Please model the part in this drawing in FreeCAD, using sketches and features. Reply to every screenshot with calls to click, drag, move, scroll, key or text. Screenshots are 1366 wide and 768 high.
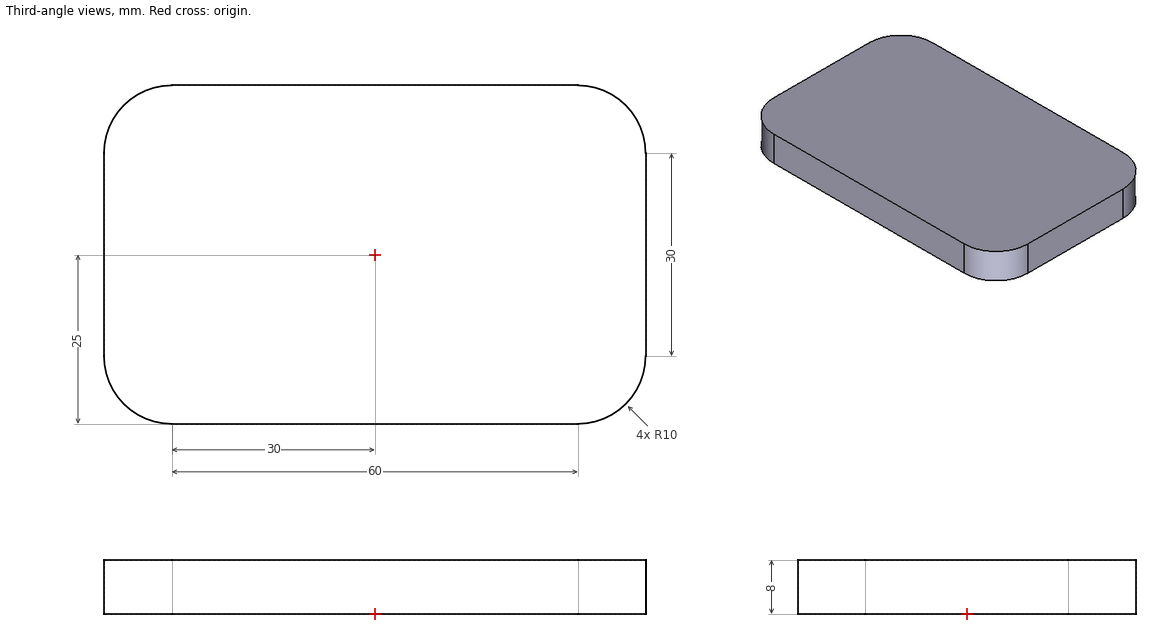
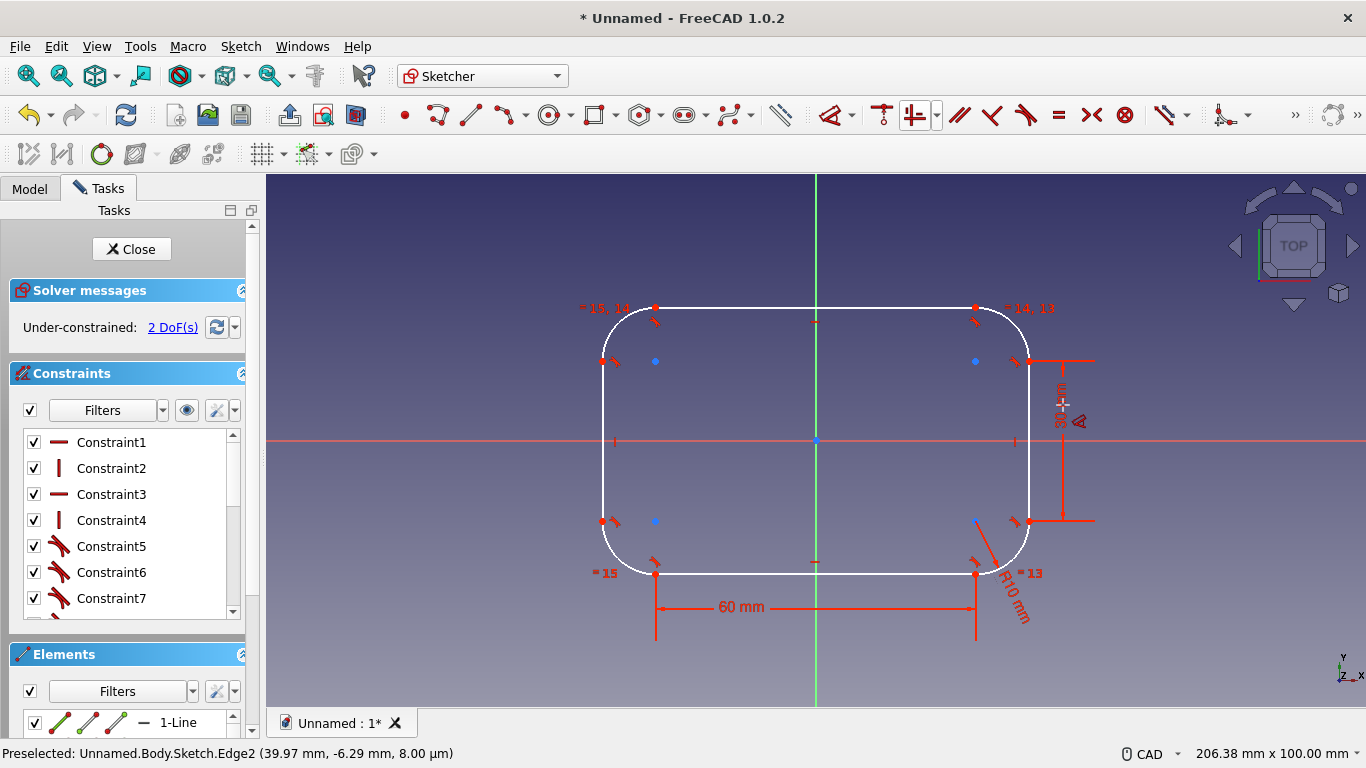
click(656, 574)
click(736, 406)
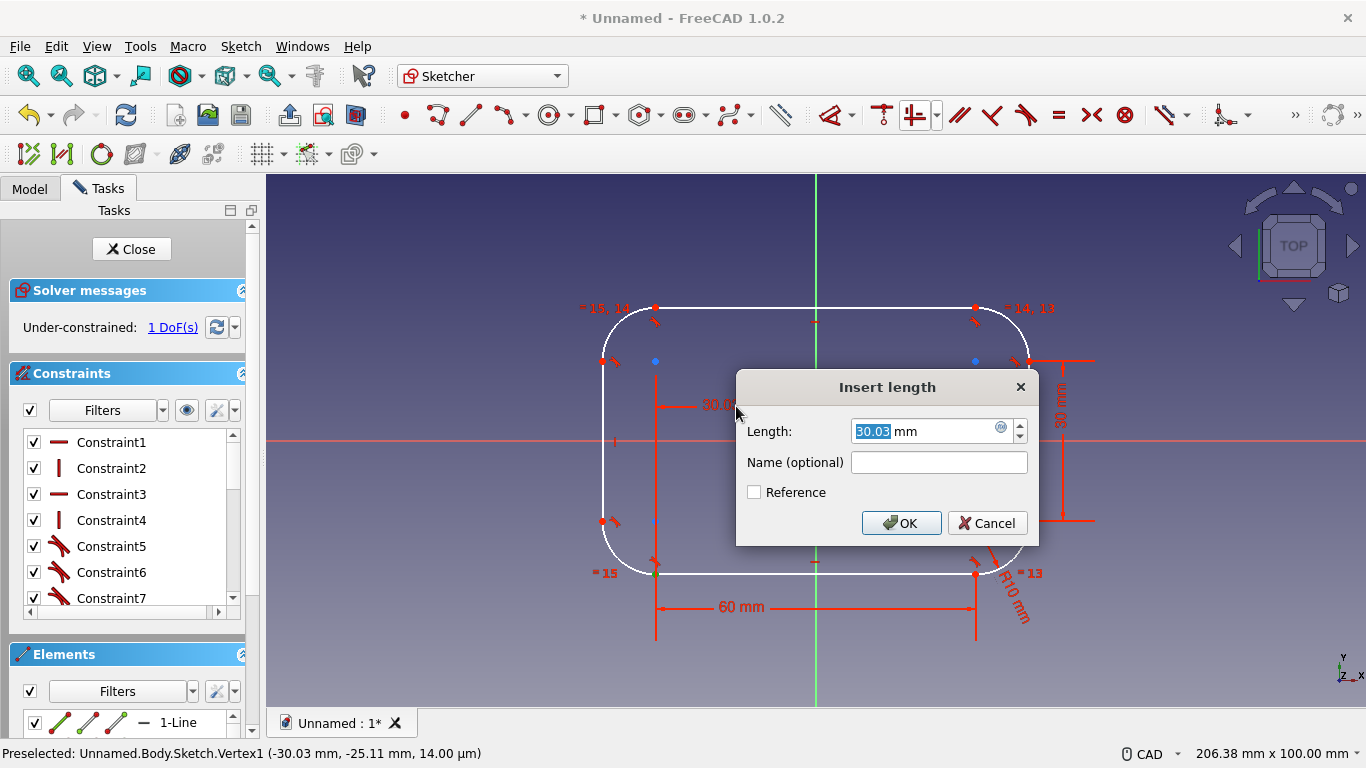
text(30)
key(Return)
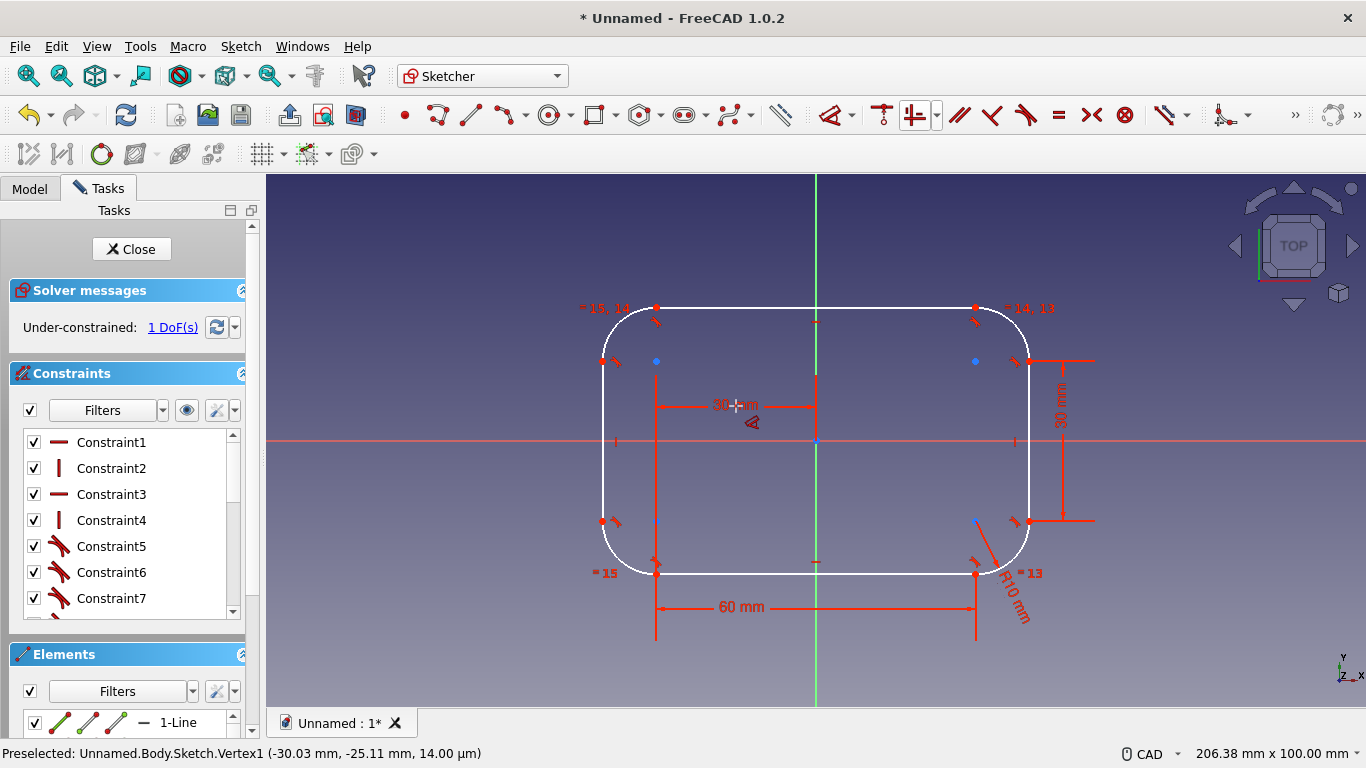
click(656, 574)
click(622, 507)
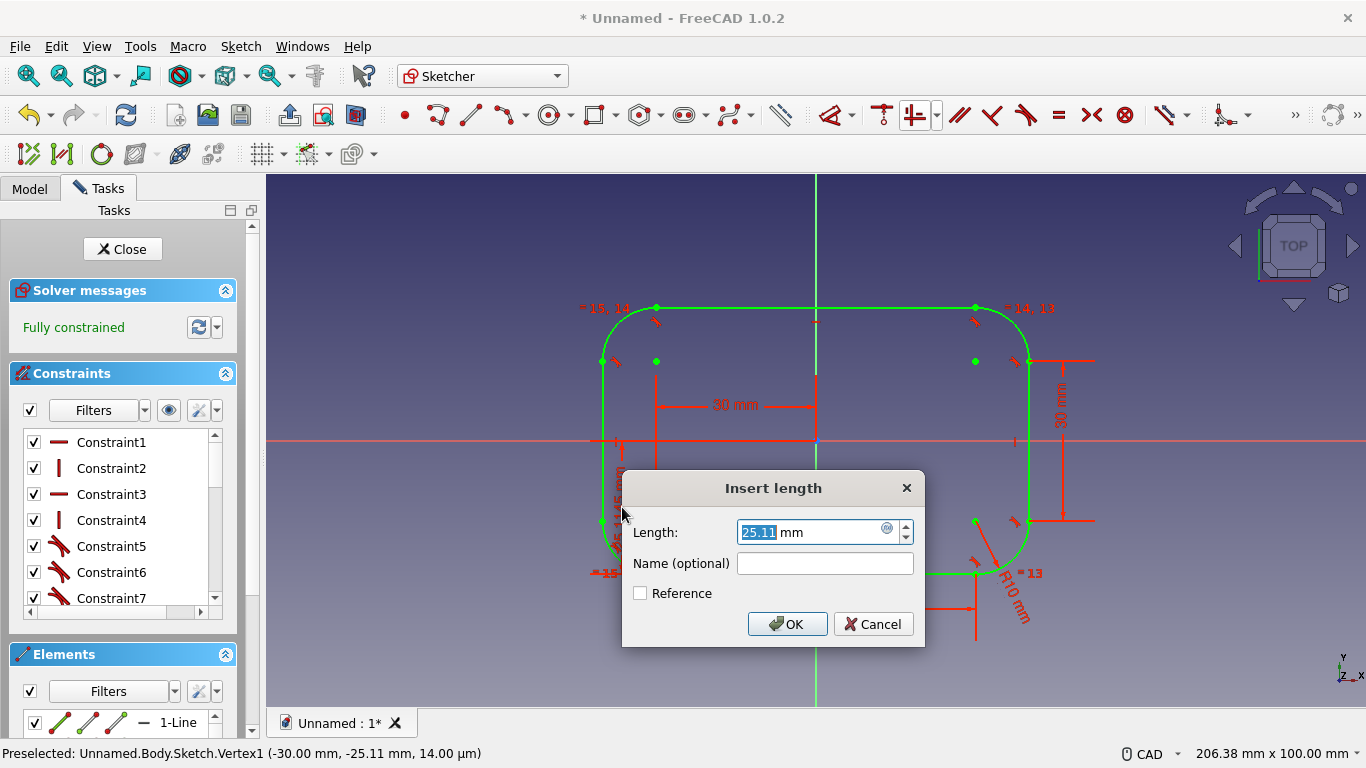
text(25)
key(Return)
key(Escape)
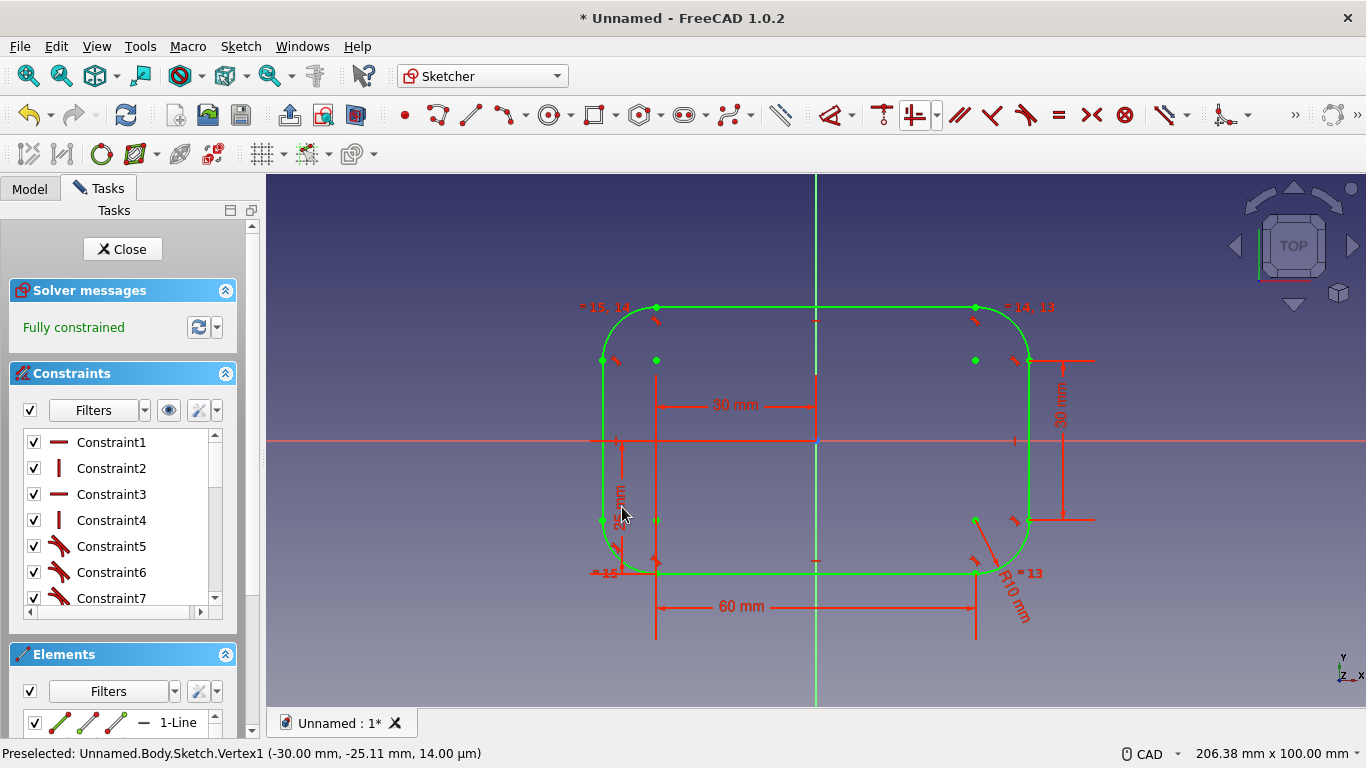
click(123, 249)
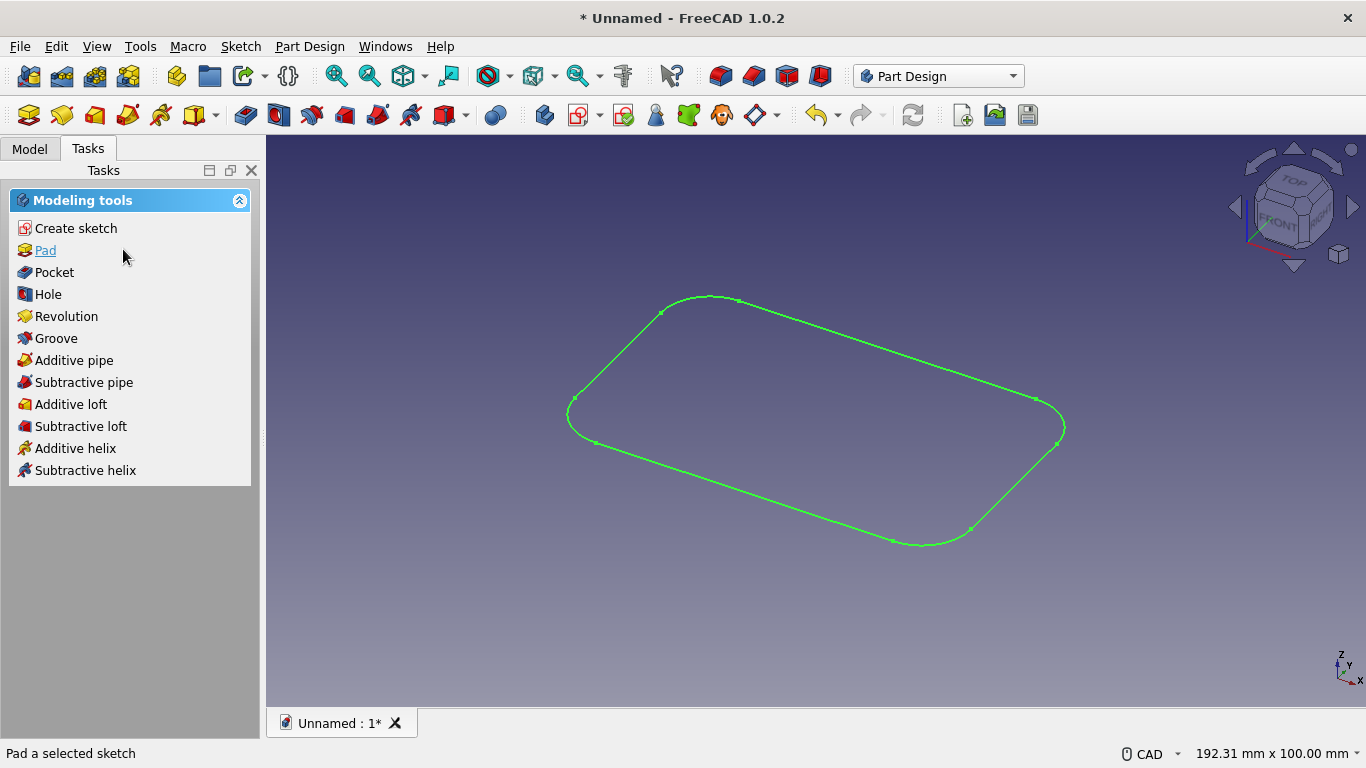
click(29, 116)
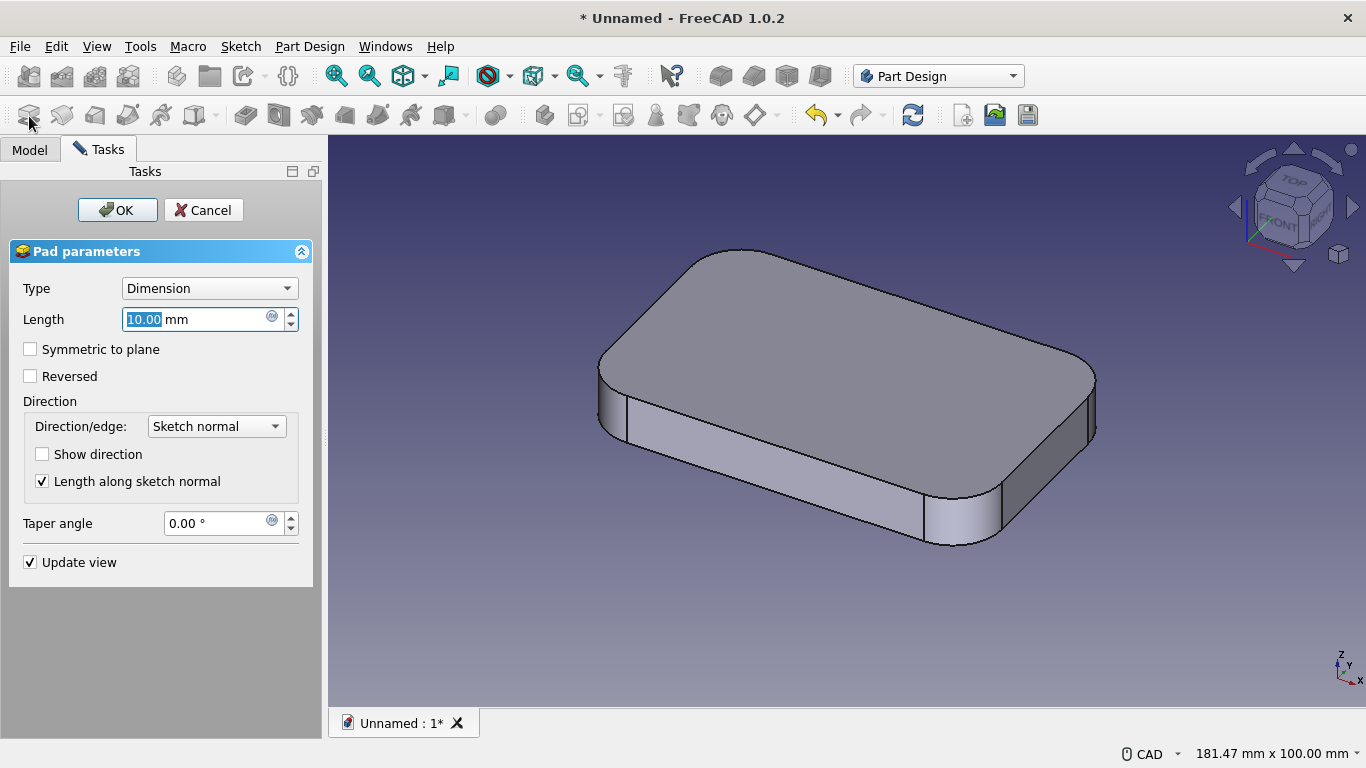
text(8)
key(Tab)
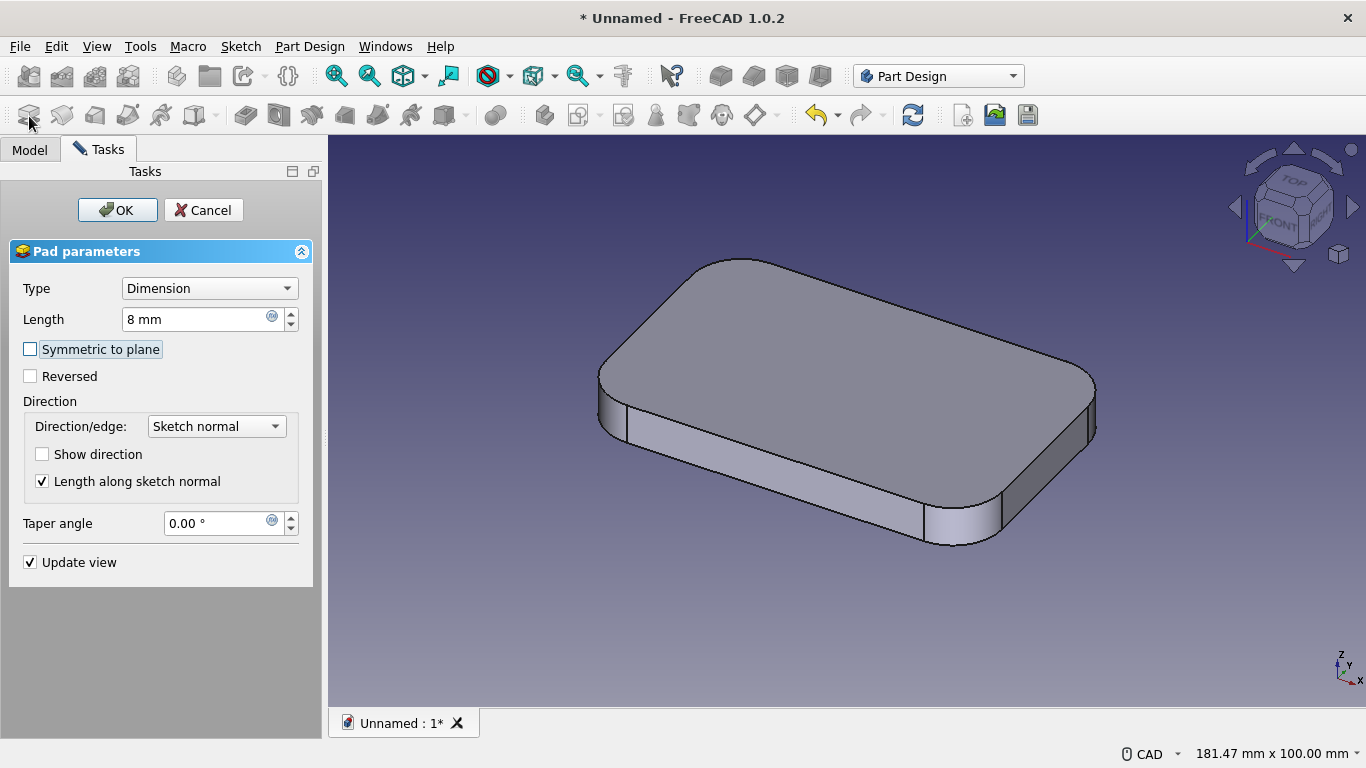
click(118, 210)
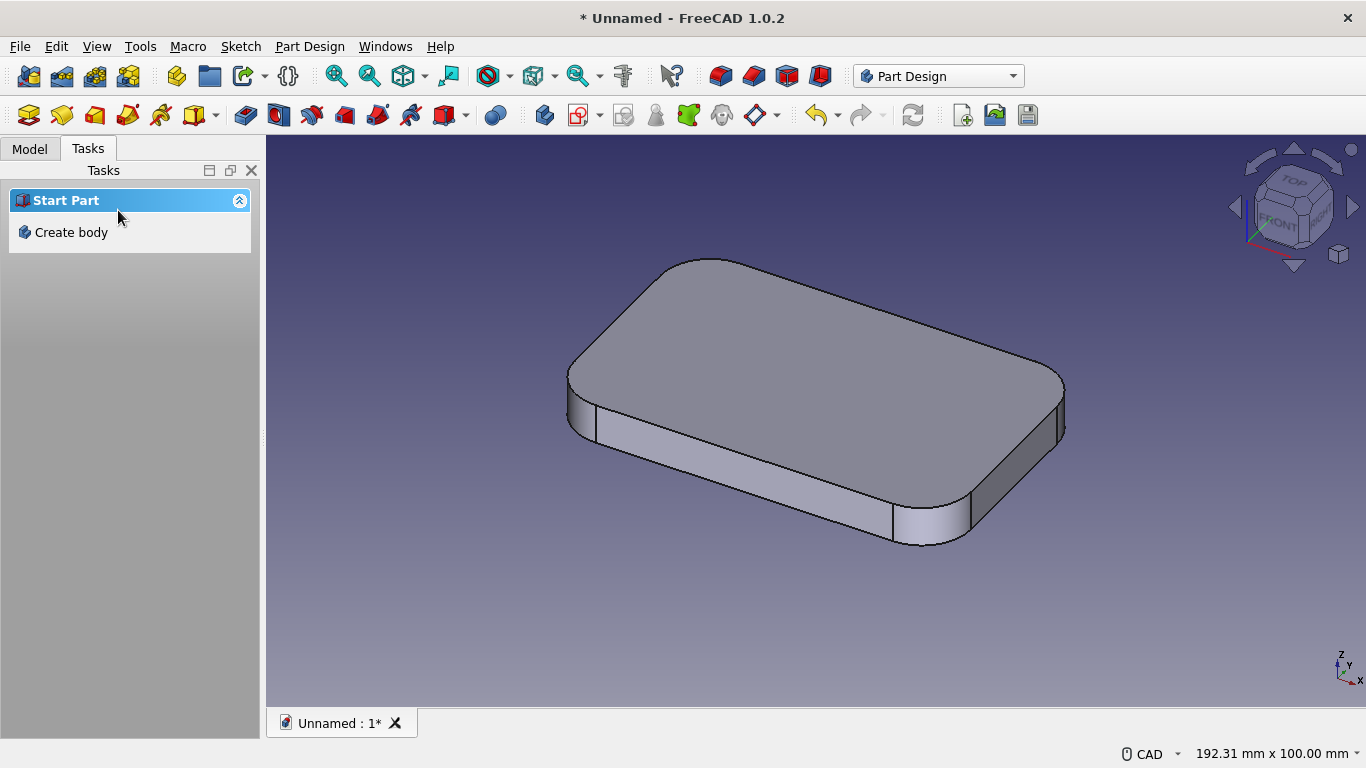
key(0)